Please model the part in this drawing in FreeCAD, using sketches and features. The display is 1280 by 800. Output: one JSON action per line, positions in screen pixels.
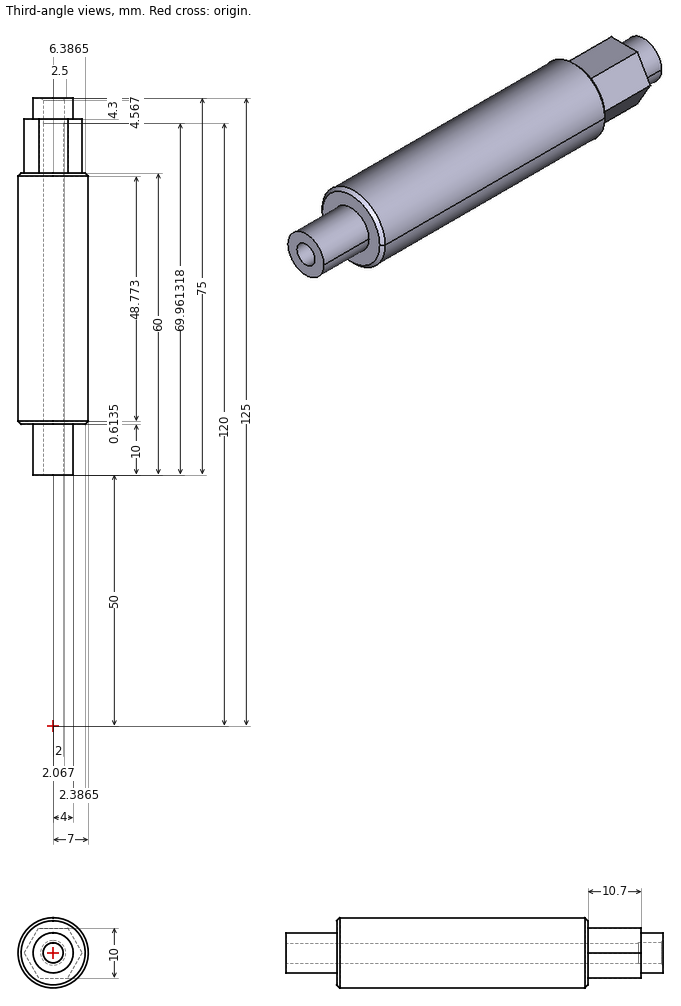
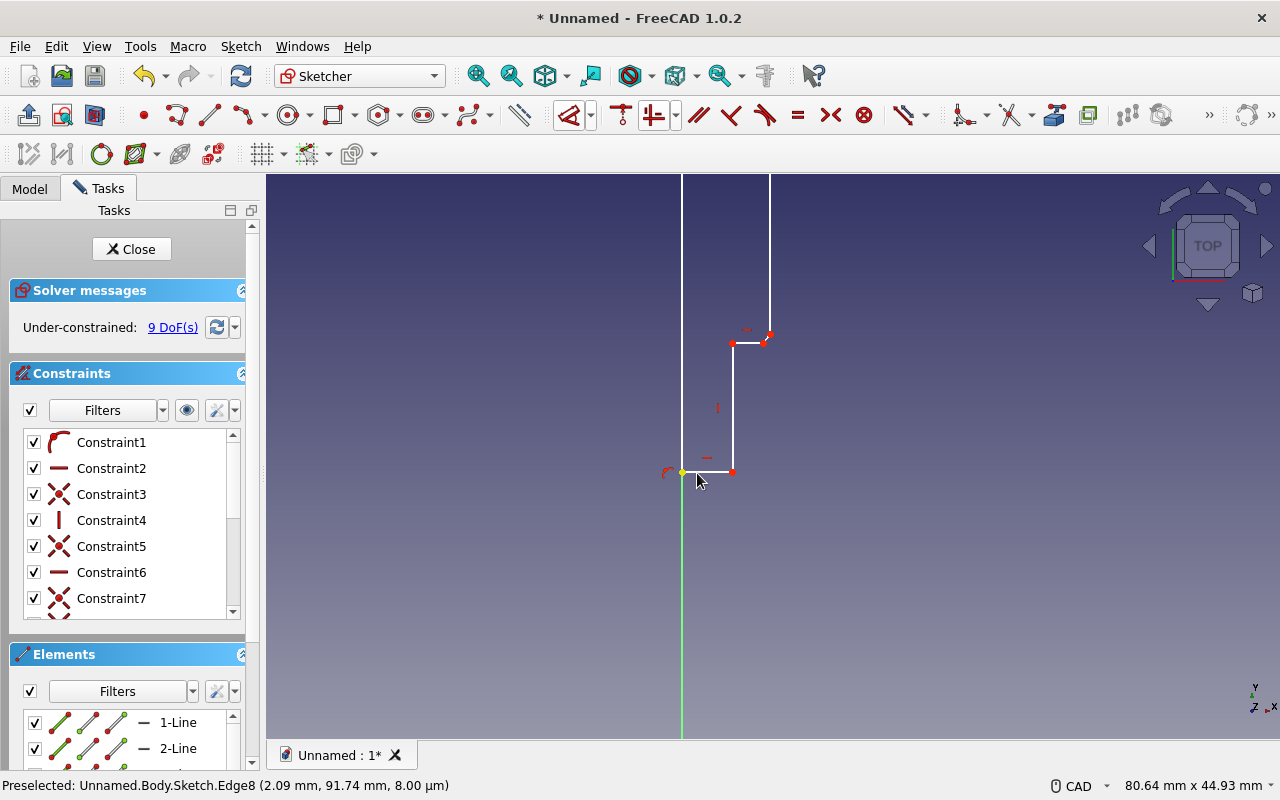
{"action": "left_click", "coordinate": [698, 472]}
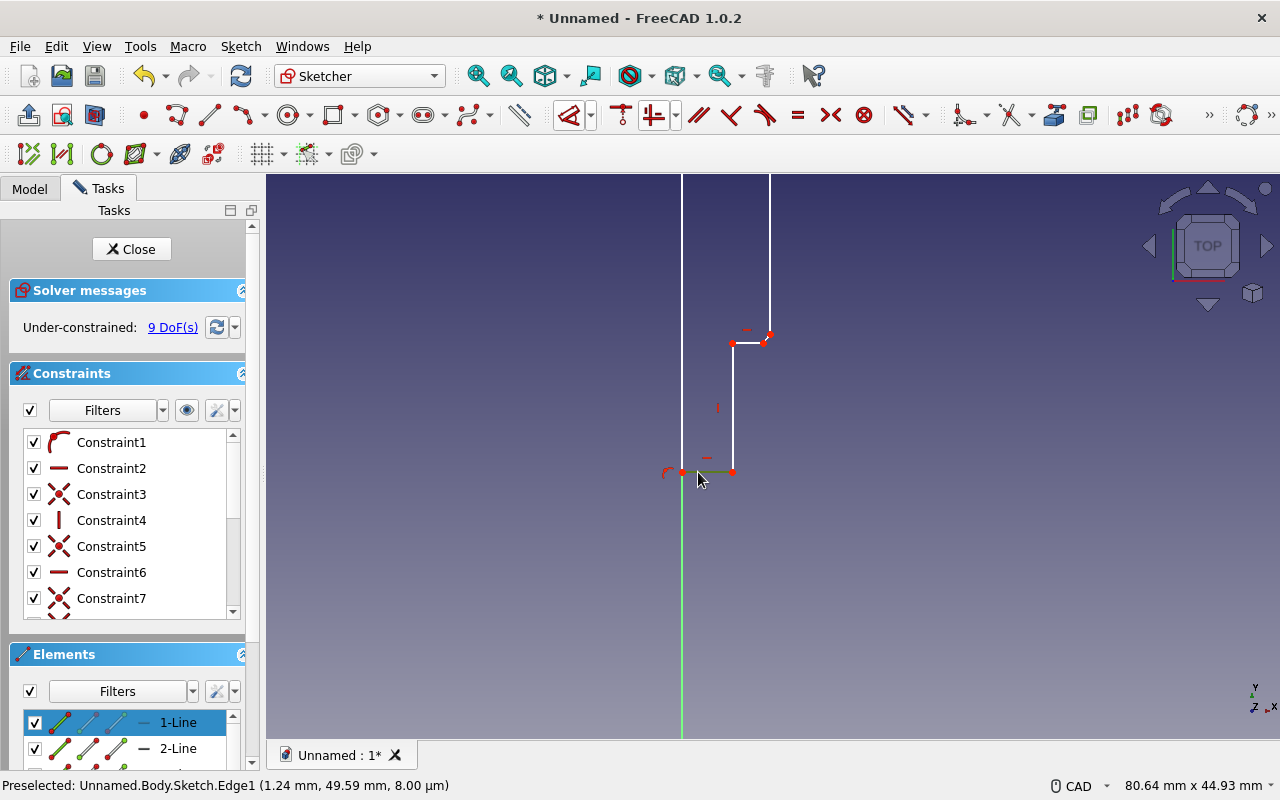
{"action": "key", "text": "l"}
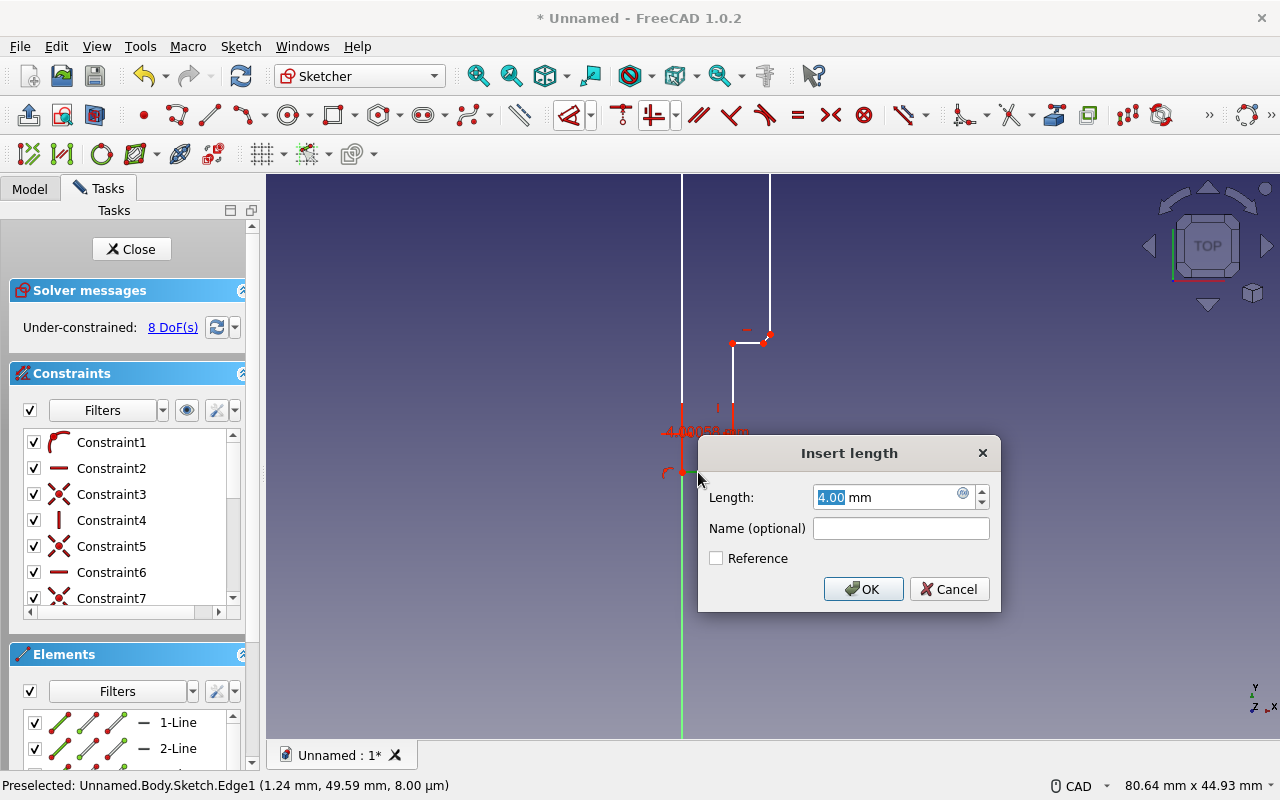
{"action": "type", "text": "4"}
{"action": "key", "text": "Return"}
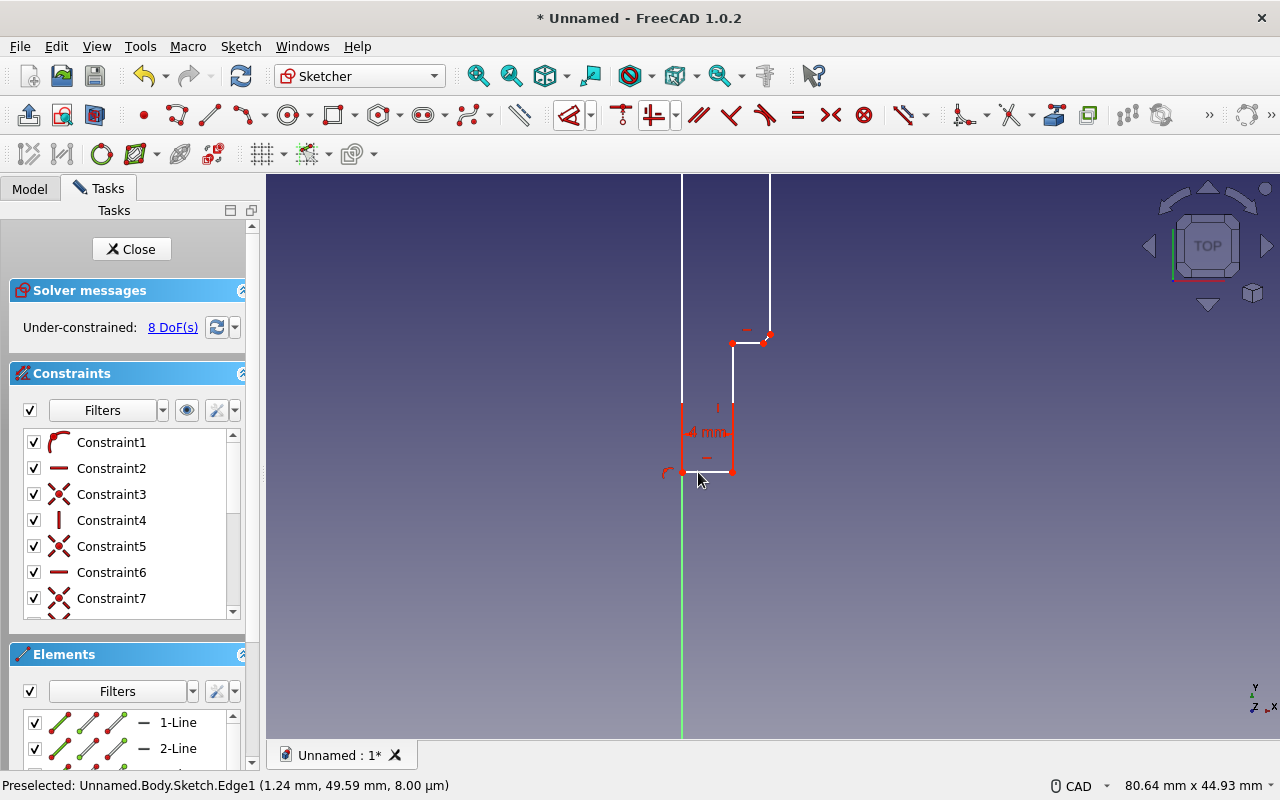
{"action": "left_click", "coordinate": [733, 433]}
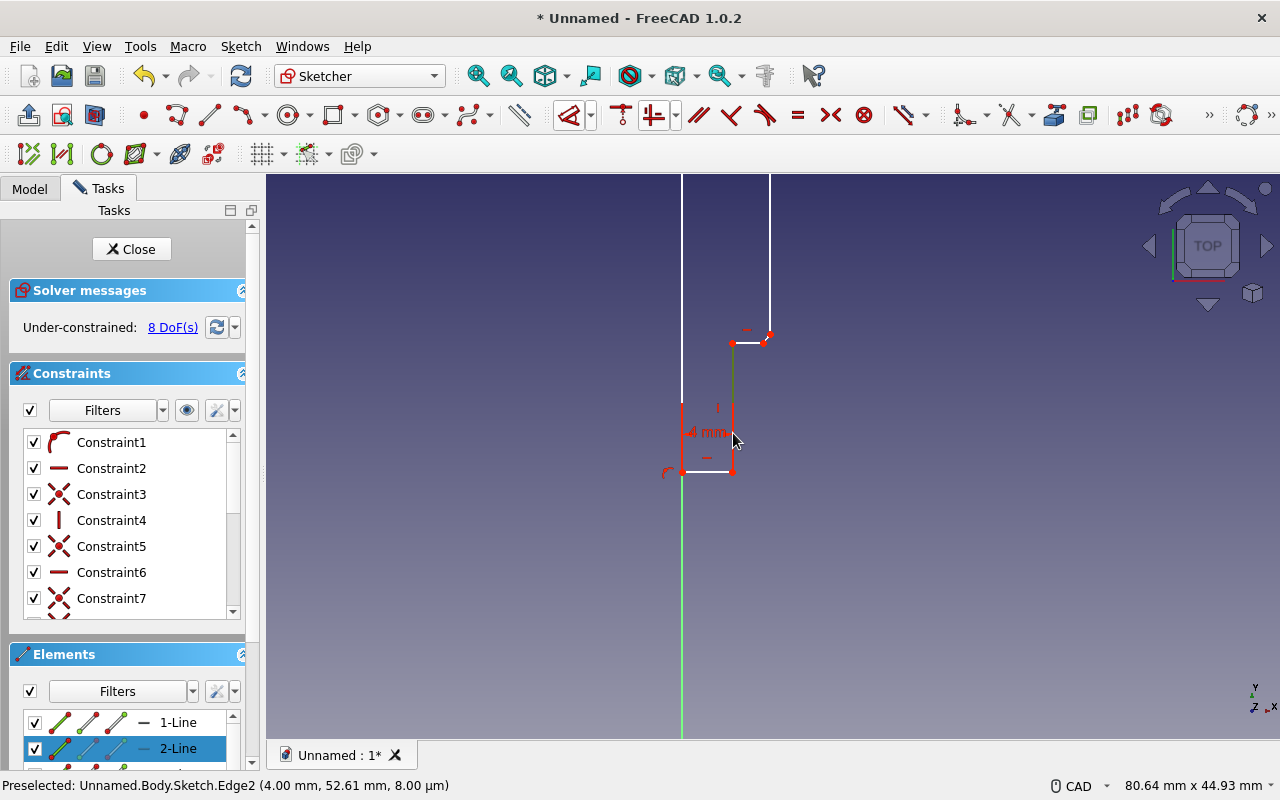
{"action": "left_click", "coordinate": [590, 116]}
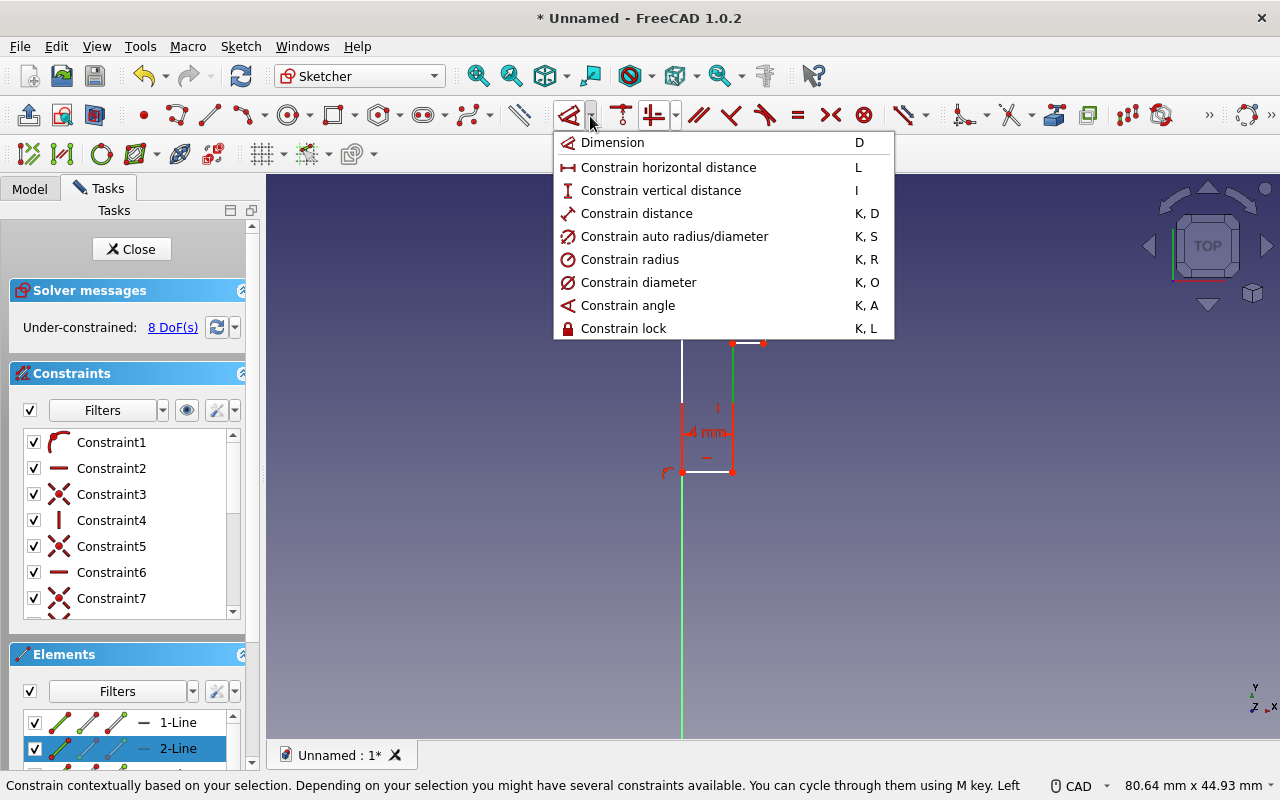
{"action": "left_click", "coordinate": [724, 190]}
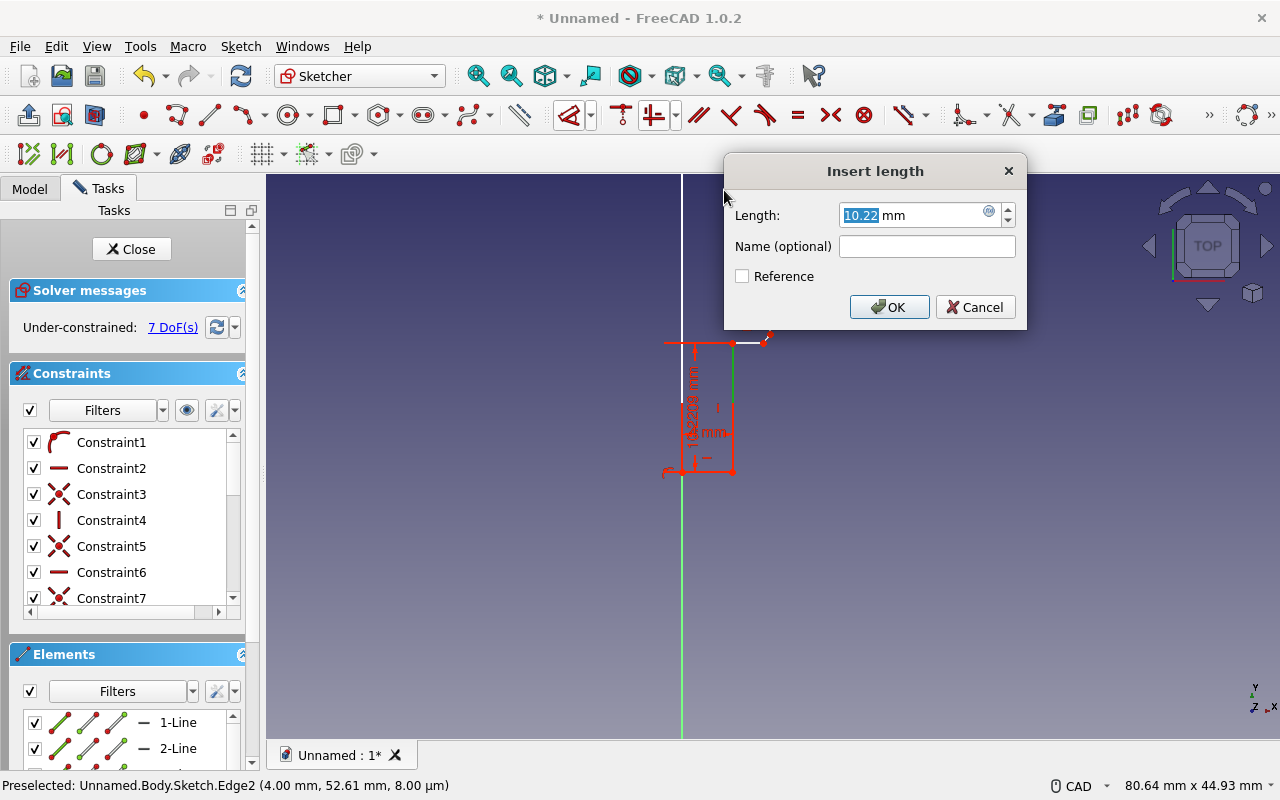
{"action": "type", "text": "10"}
{"action": "key", "text": "Return"}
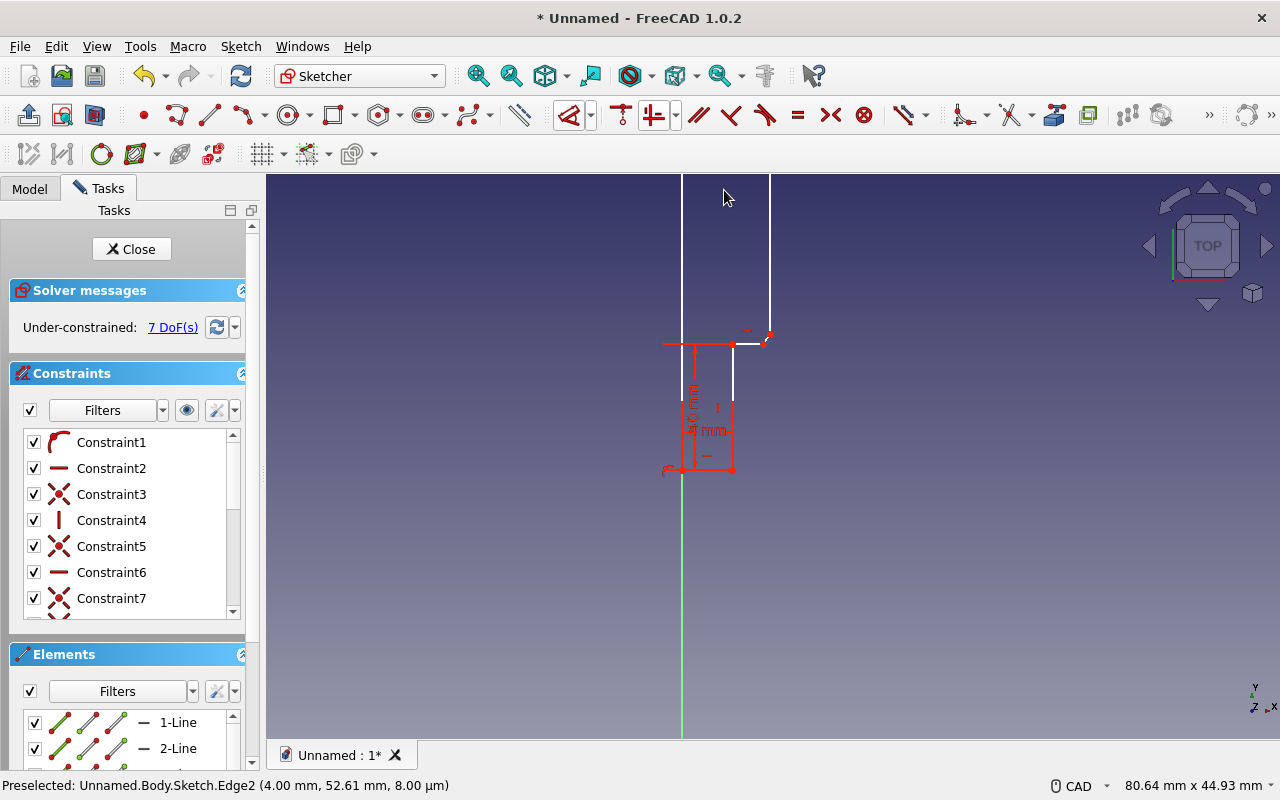
{"action": "scroll", "coordinate": [697, 474], "scroll_direction": "down", "scroll_amount": 7}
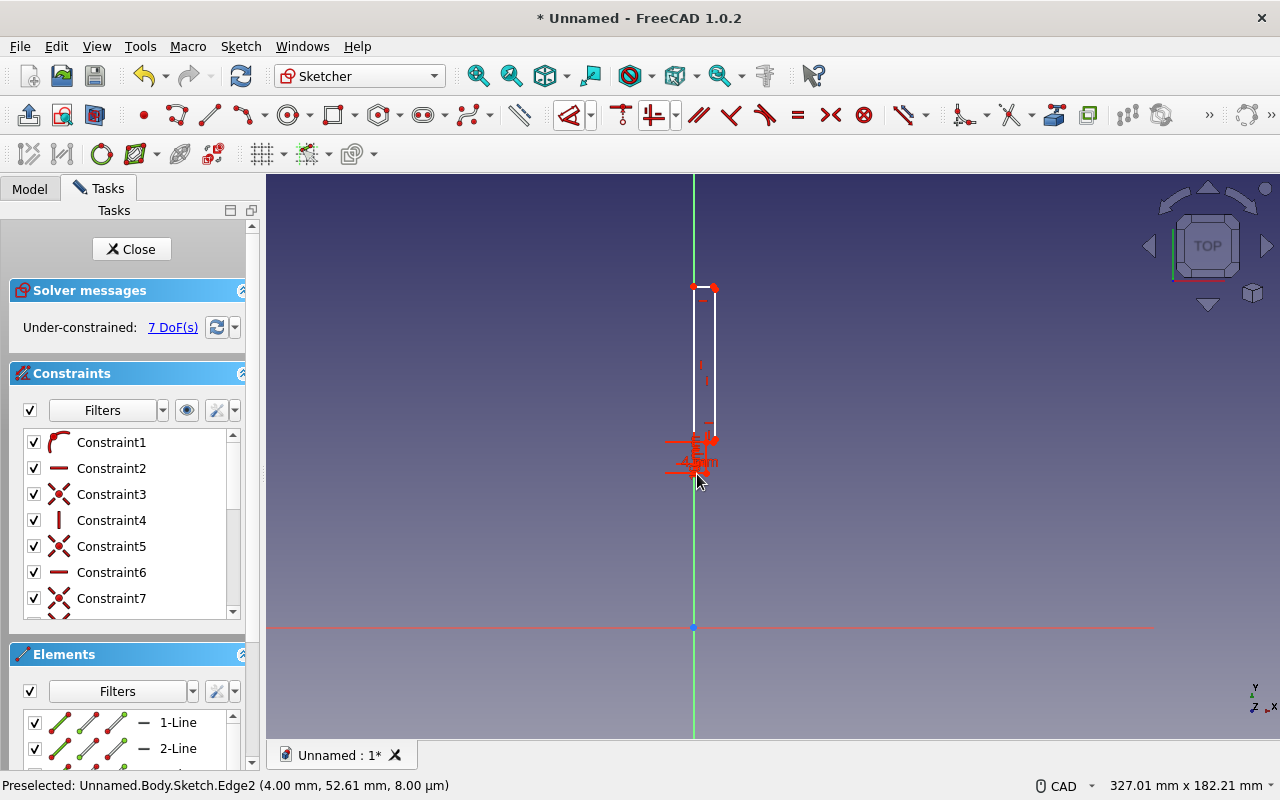
{"action": "left_click", "coordinate": [694, 417]}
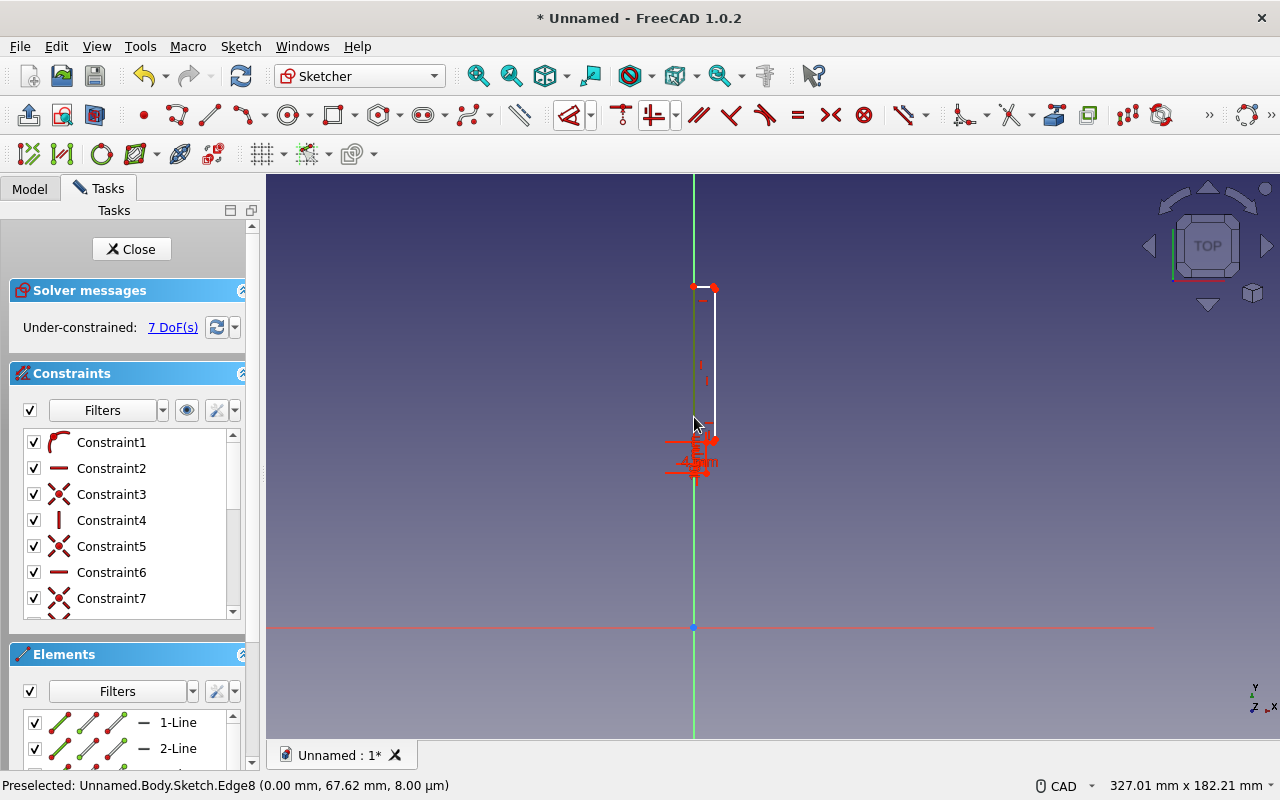
{"action": "key", "text": "i"}